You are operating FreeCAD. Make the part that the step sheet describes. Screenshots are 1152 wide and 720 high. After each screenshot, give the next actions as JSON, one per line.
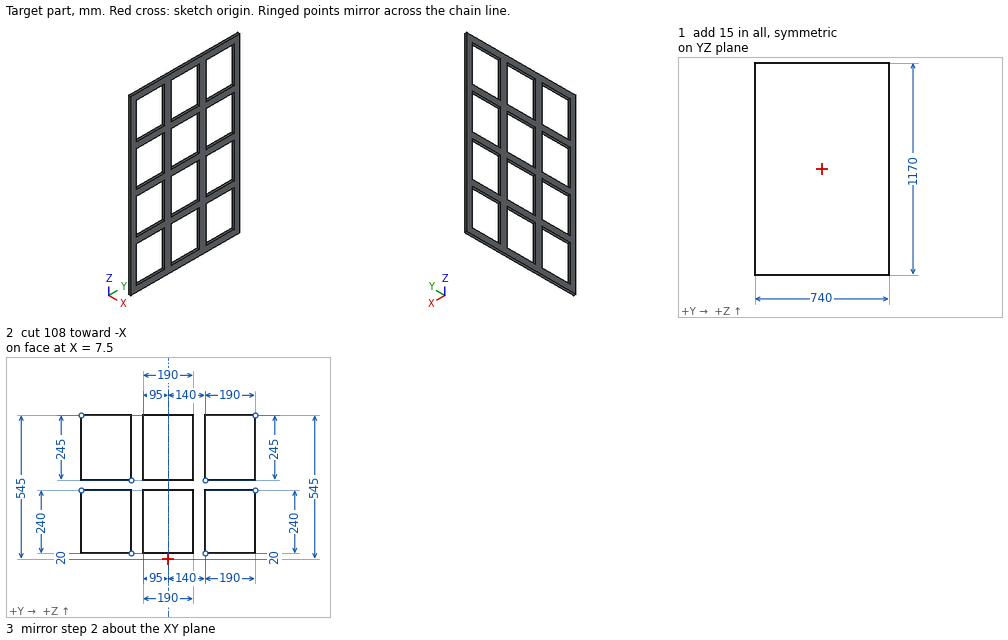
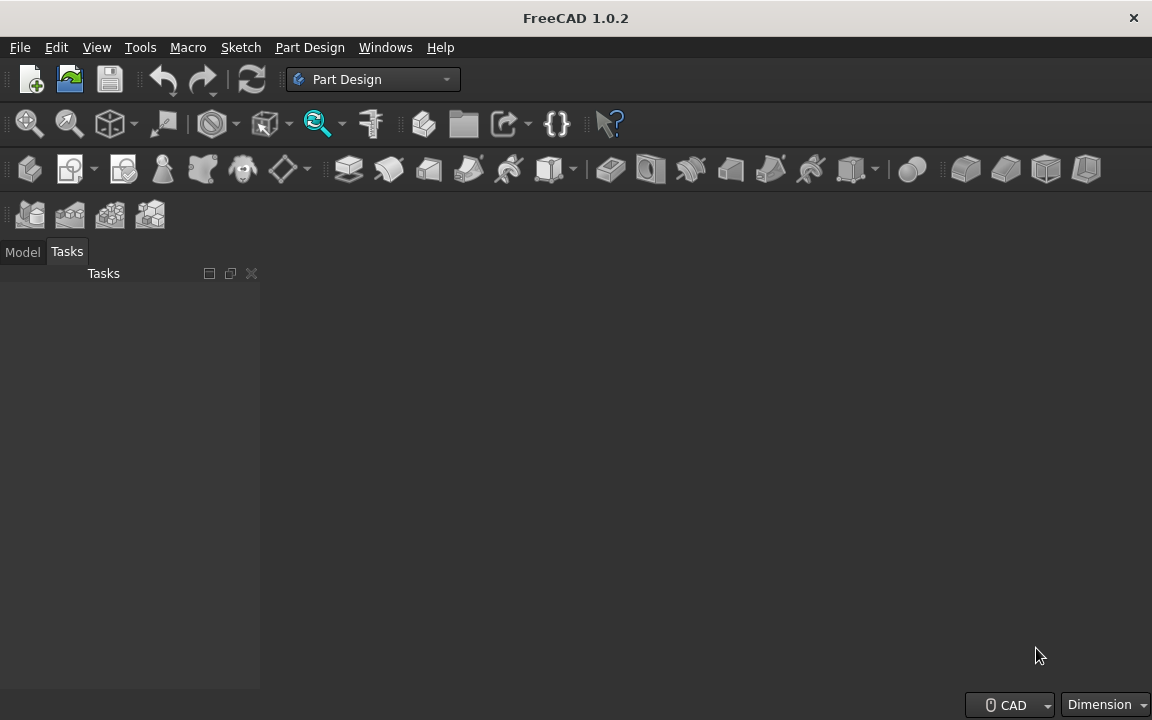
{"action": "left_click", "coordinate": [30, 80]}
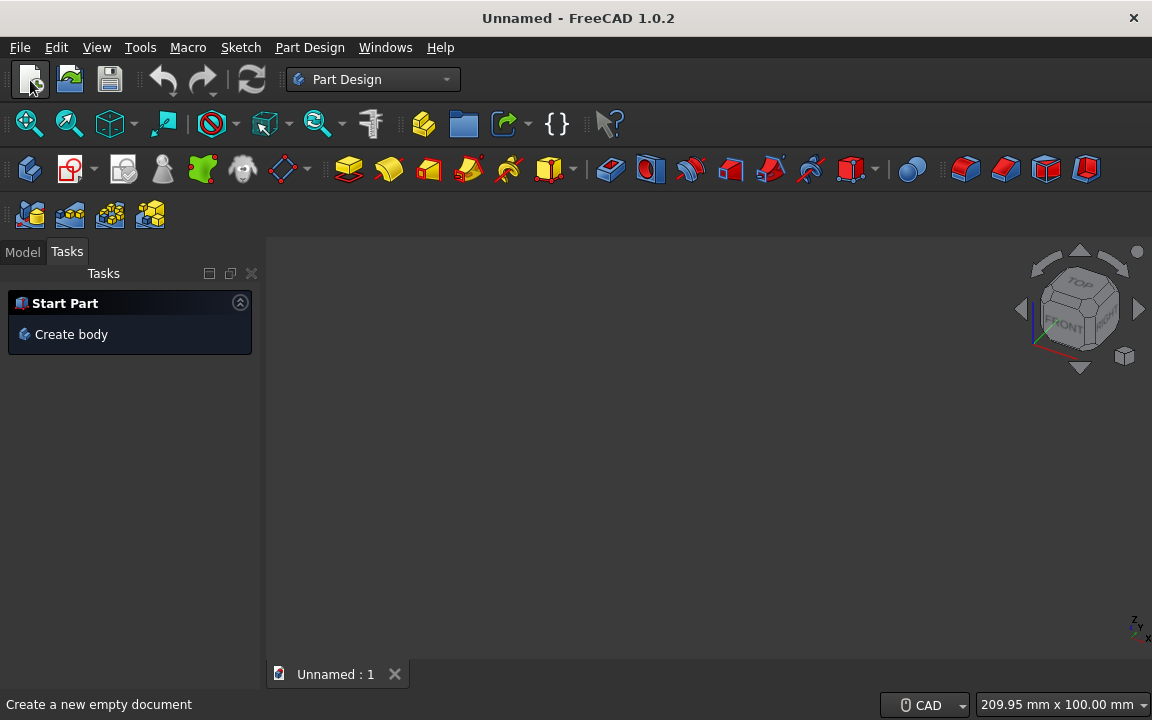
{"action": "left_click", "coordinate": [70, 170]}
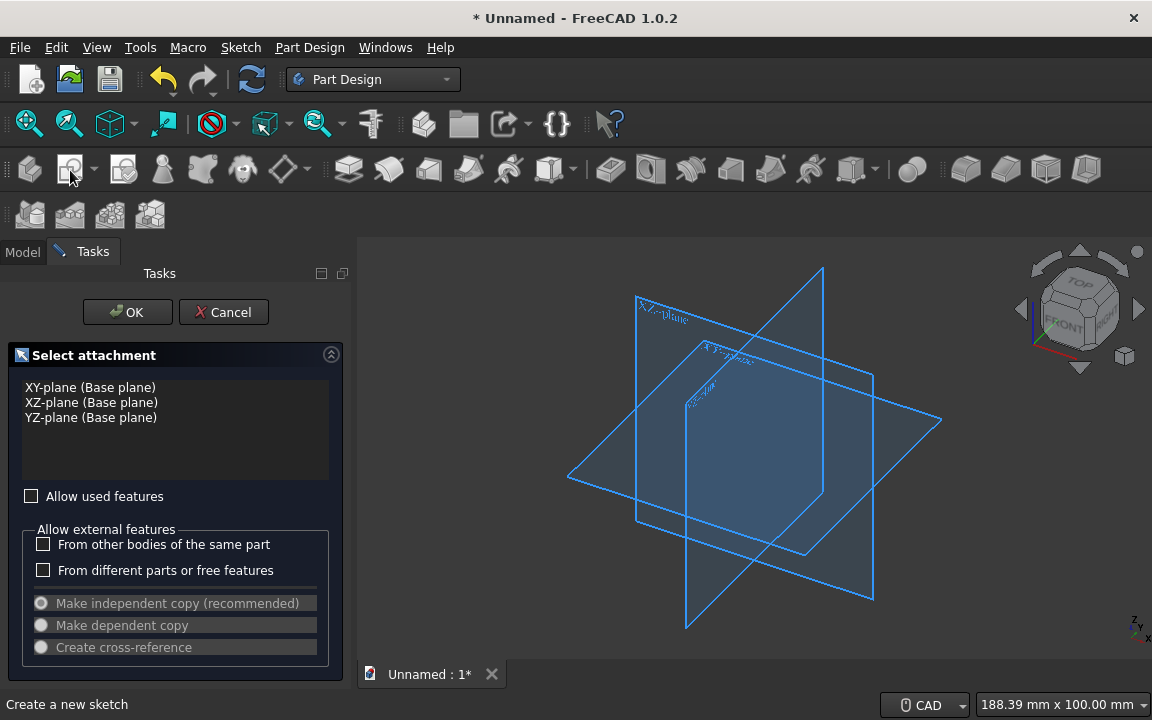
{"action": "left_click", "coordinate": [82, 418]}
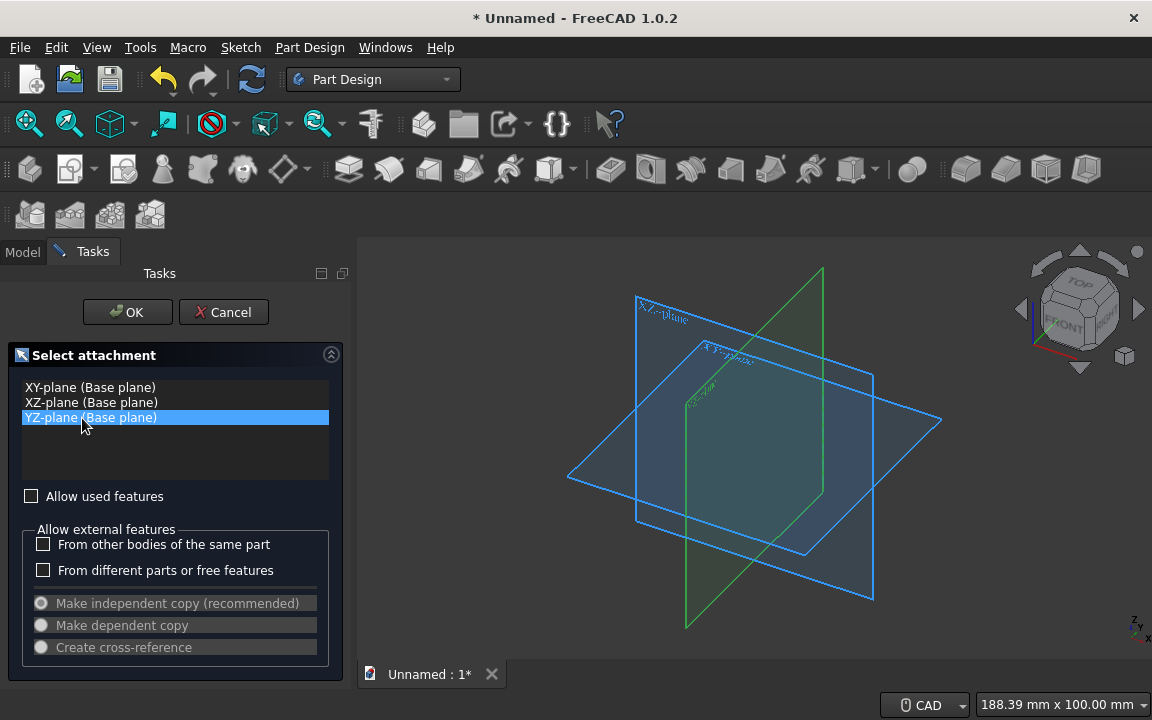
{"action": "left_click", "coordinate": [128, 312]}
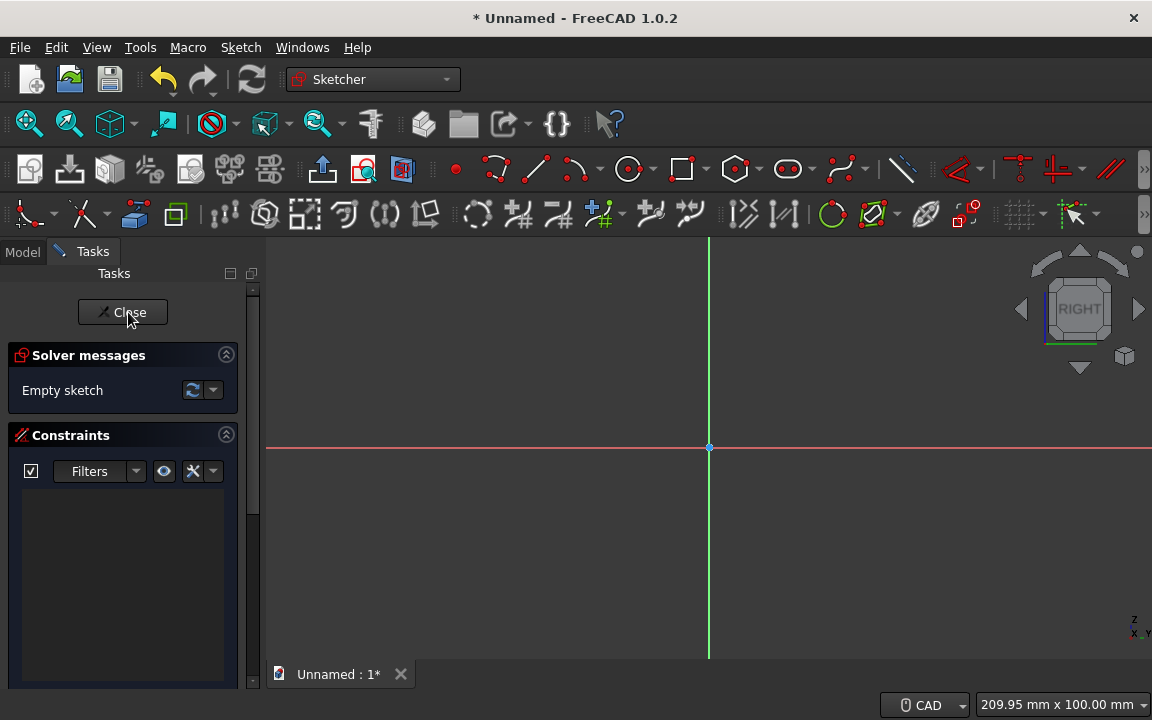
{"action": "scroll", "coordinate": [637, 448], "scroll_direction": "down", "scroll_amount": 15}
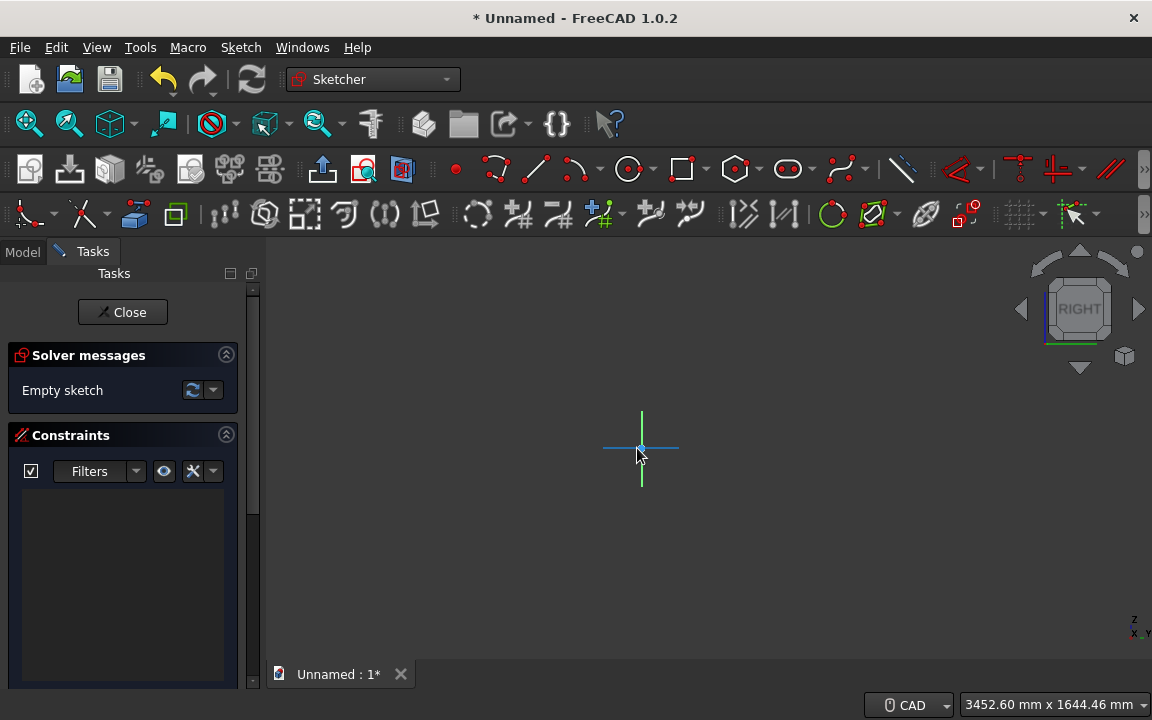
{"action": "key", "text": "g v"}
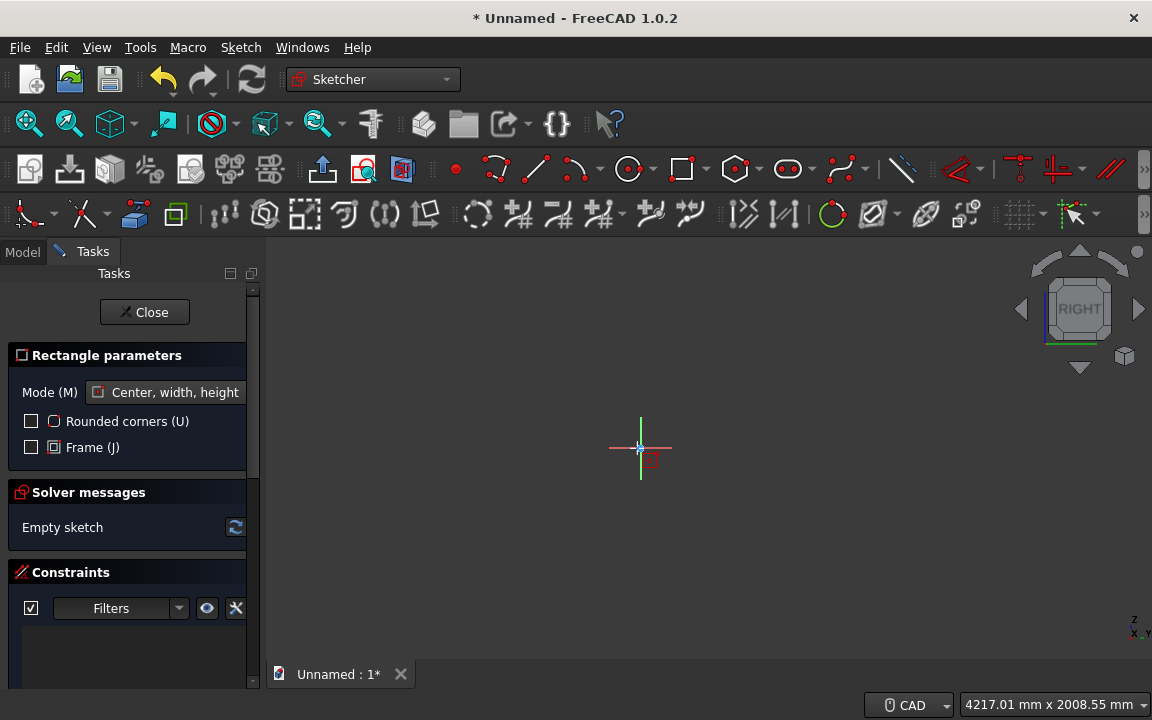
{"action": "left_click", "coordinate": [641, 448]}
{"action": "left_click", "coordinate": [719, 326]}
{"action": "key", "text": "Escape"}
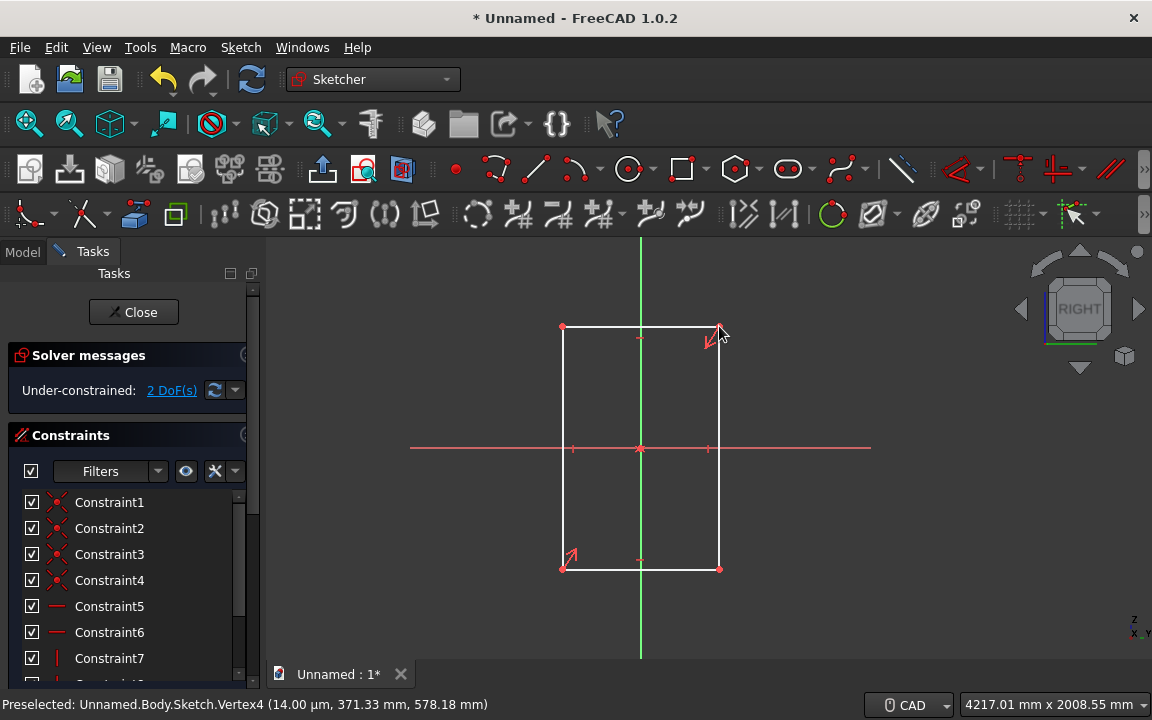
{"action": "left_click", "coordinate": [956, 170]}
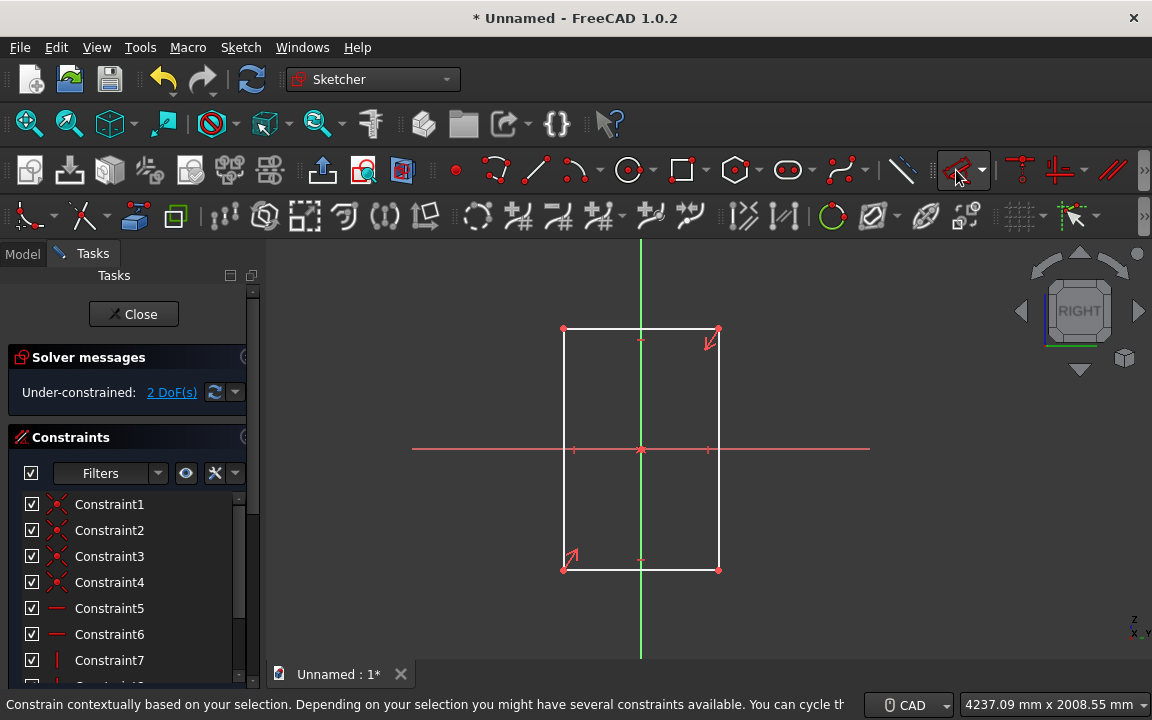
{"action": "left_click", "coordinate": [610, 570]}
{"action": "left_click", "coordinate": [606, 604]}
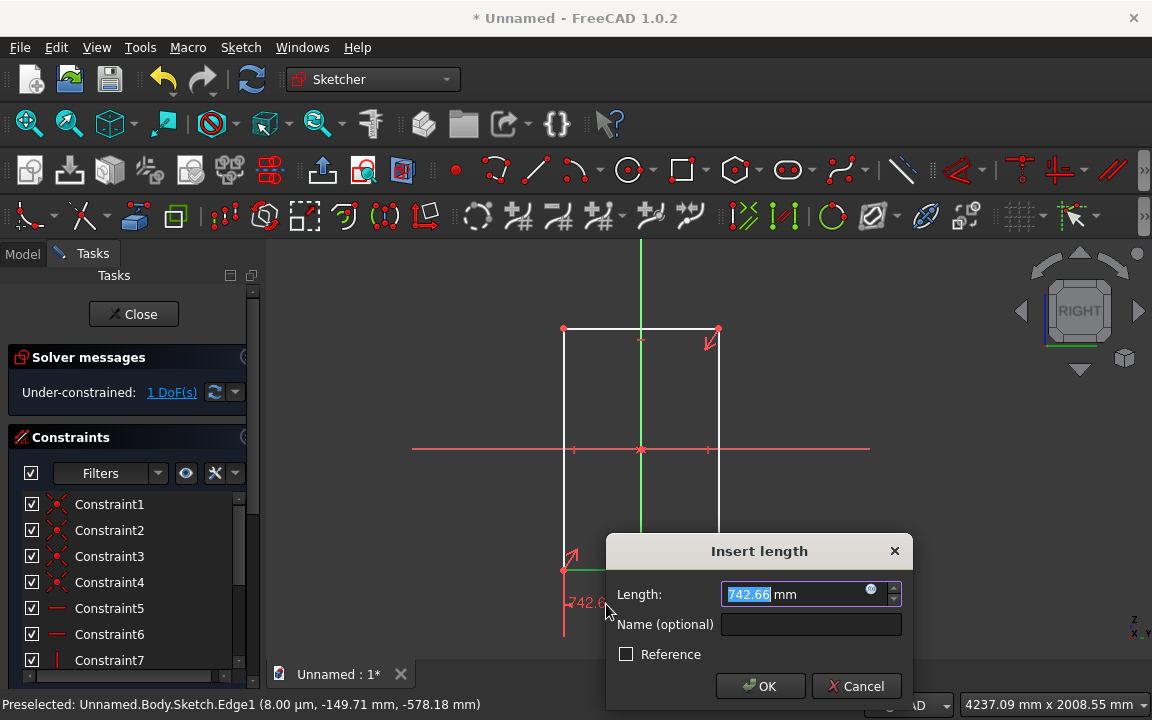
{"action": "type", "text": "740"}
{"action": "key", "text": "Return"}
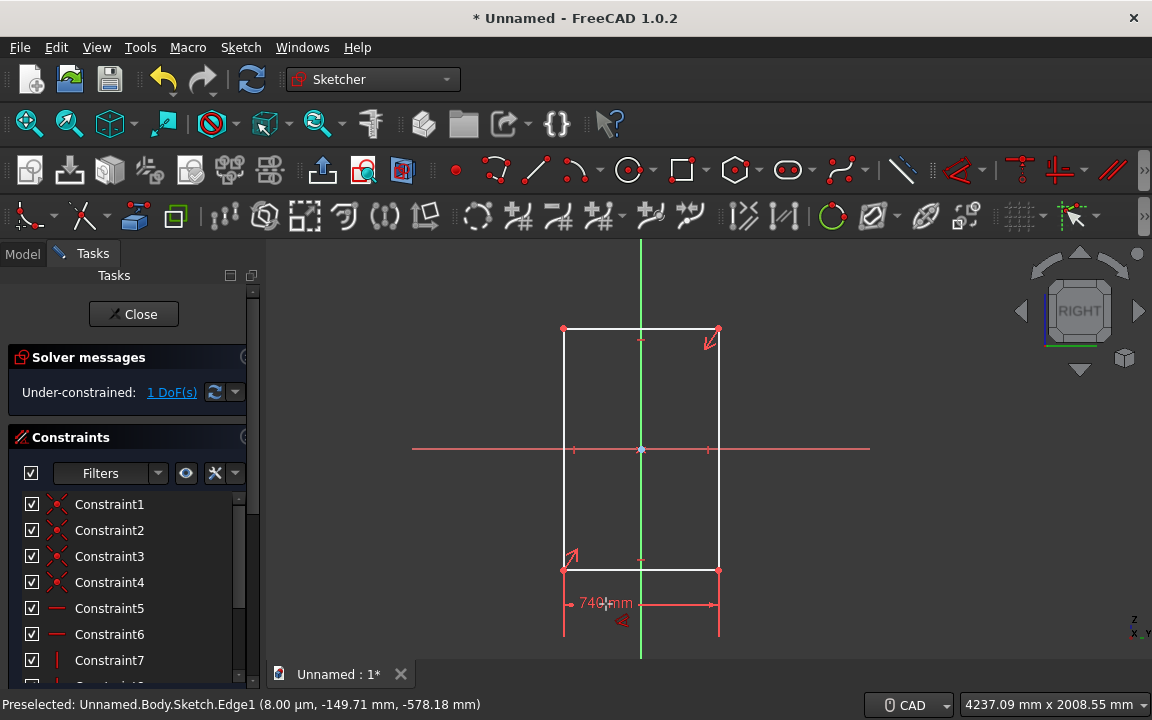
{"action": "left_click", "coordinate": [719, 498]}
{"action": "left_click", "coordinate": [753, 394]}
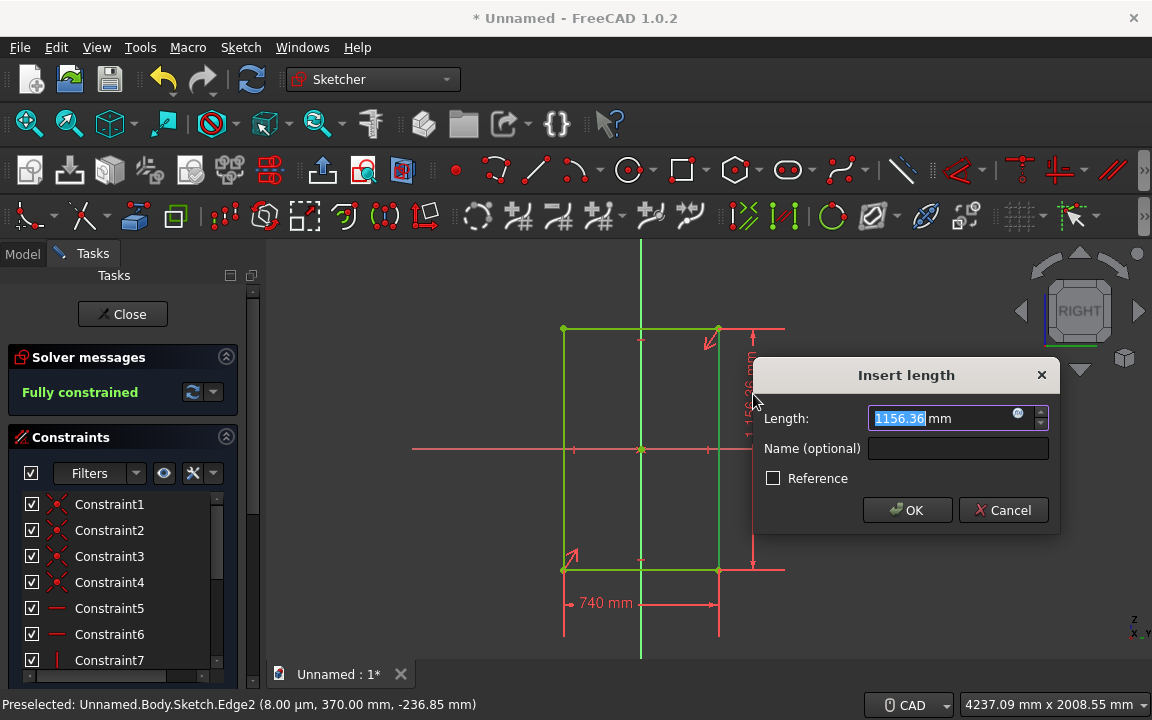
{"action": "type", "text": "1170"}
{"action": "key", "text": "Return"}
{"action": "key", "text": "Escape"}